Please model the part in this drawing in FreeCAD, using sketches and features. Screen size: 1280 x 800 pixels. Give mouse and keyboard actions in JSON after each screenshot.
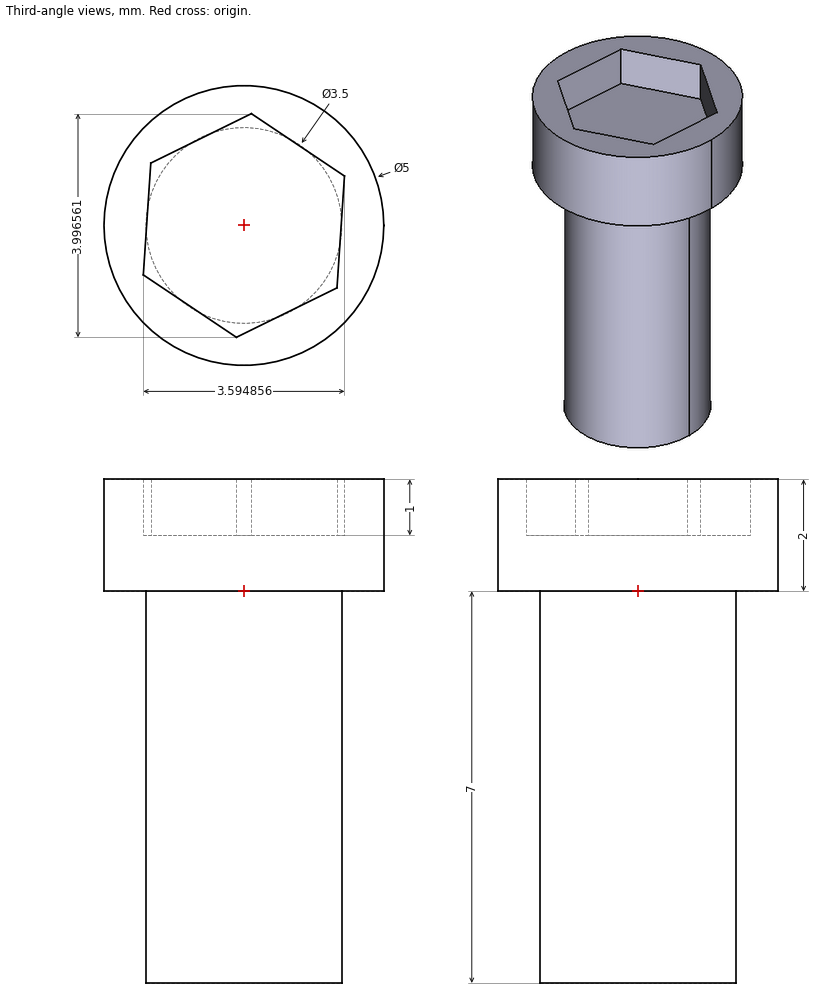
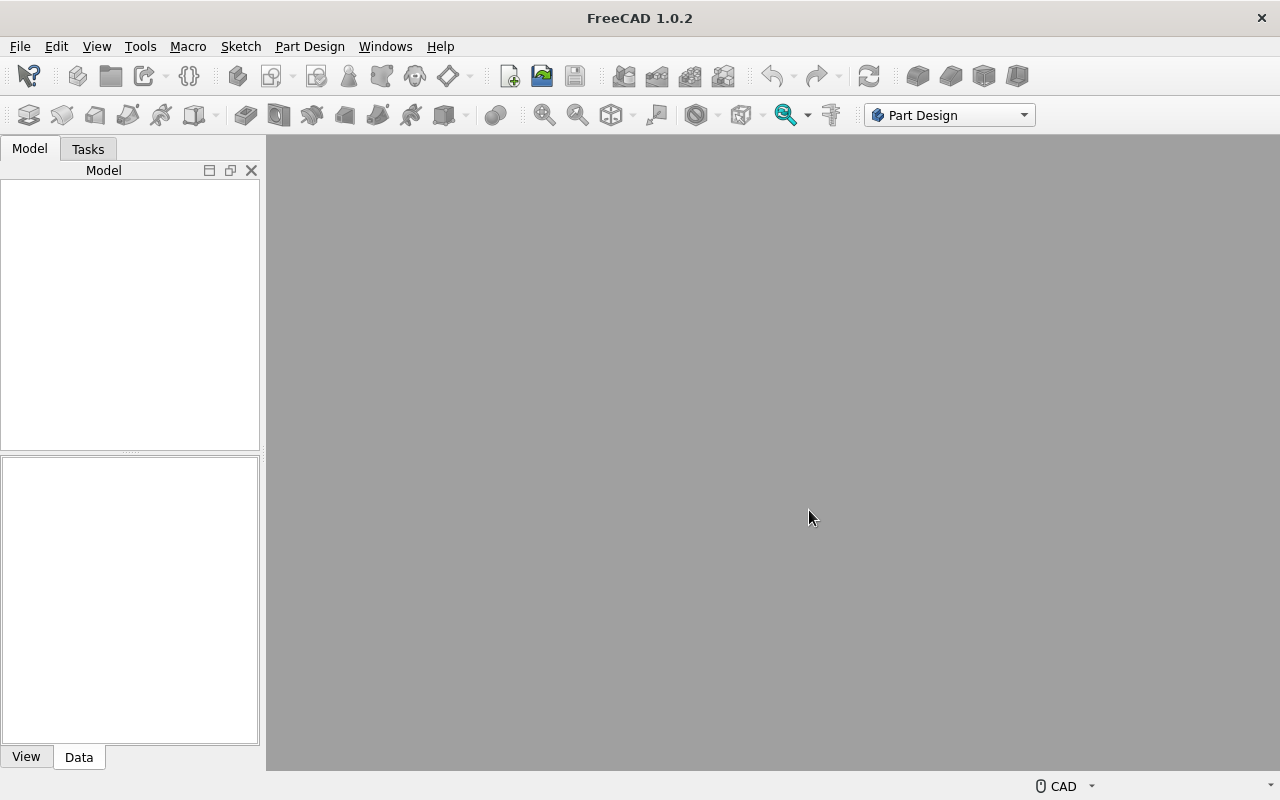
{"action": "left_click", "coordinate": [509, 76]}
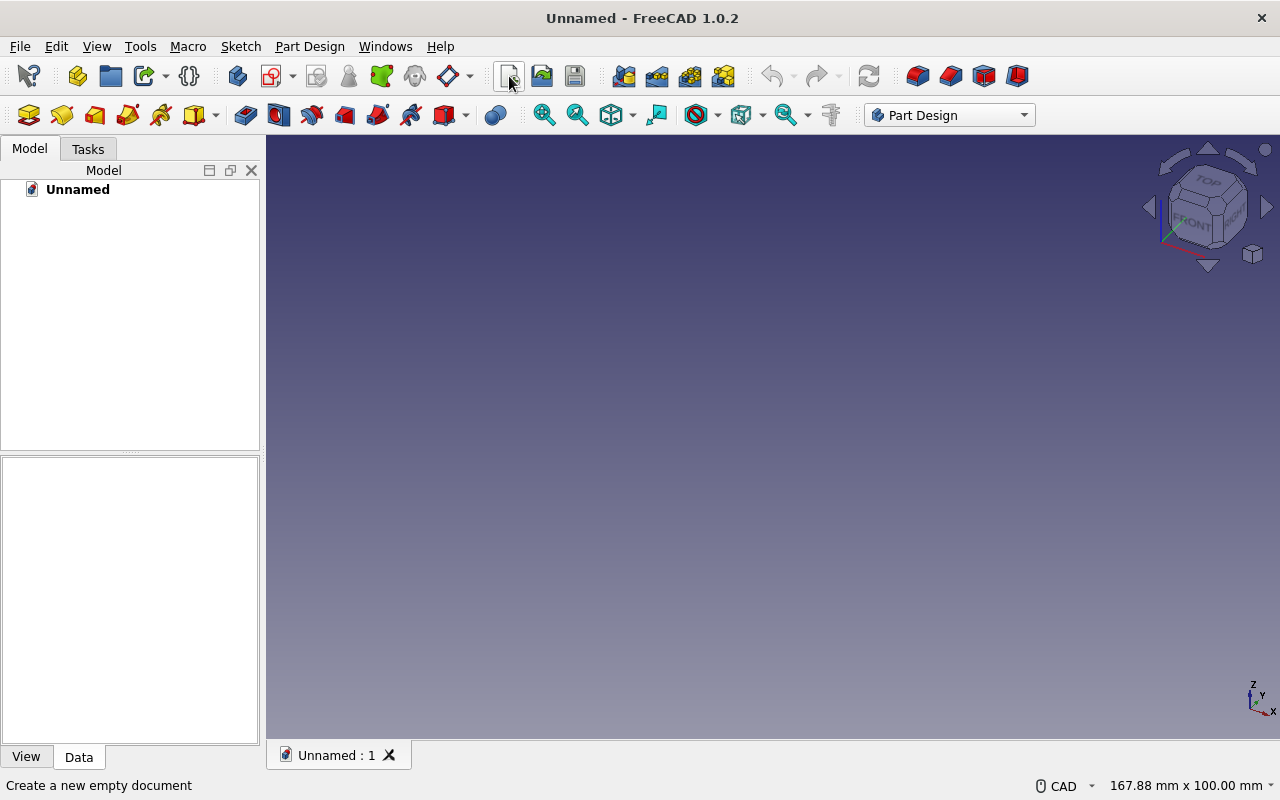
{"action": "left_click", "coordinate": [270, 76]}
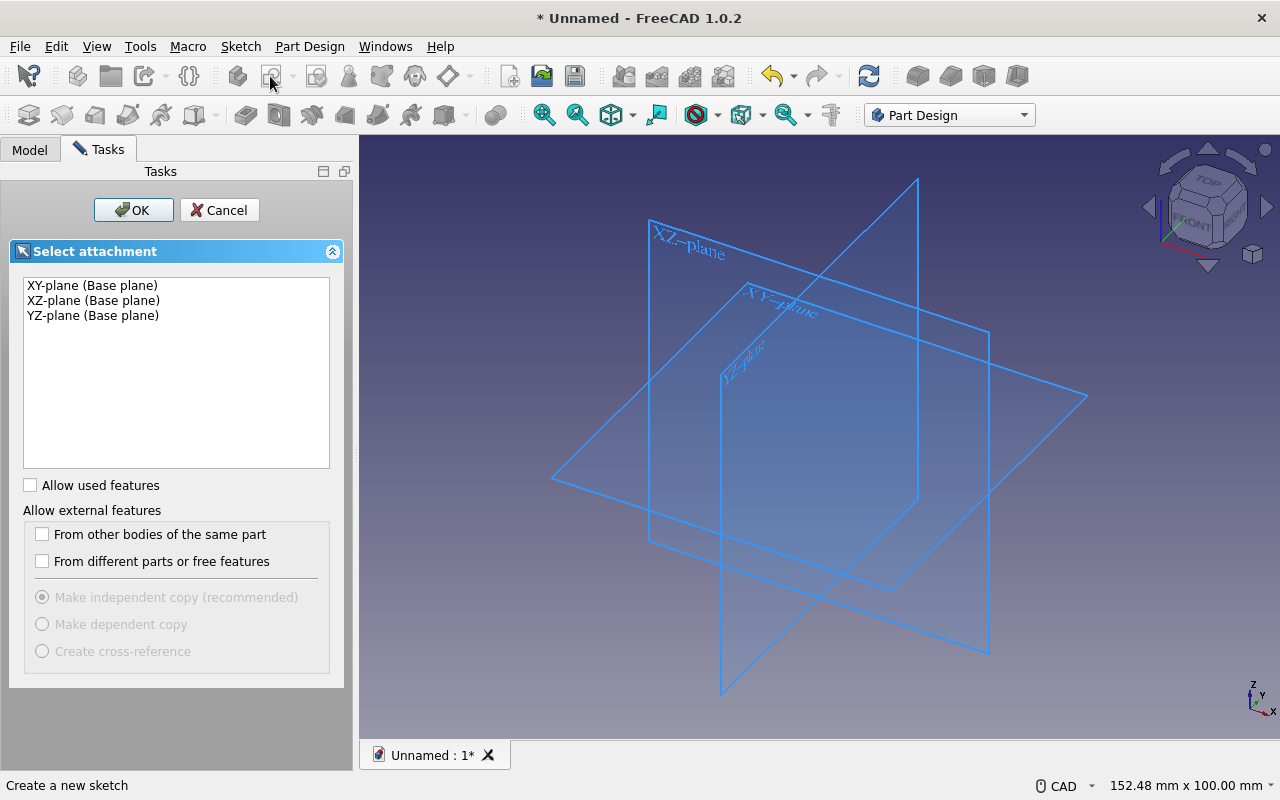
{"action": "left_click", "coordinate": [84, 286]}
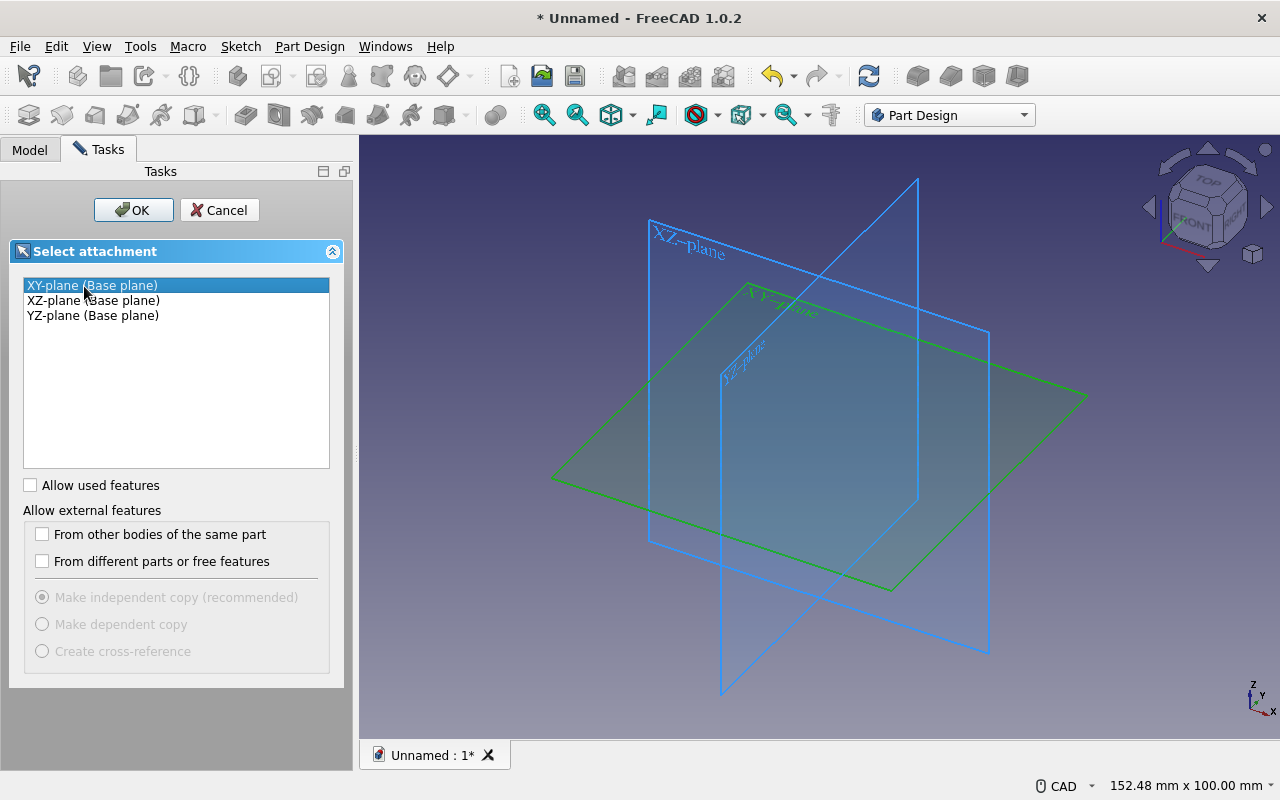
{"action": "left_click", "coordinate": [134, 210]}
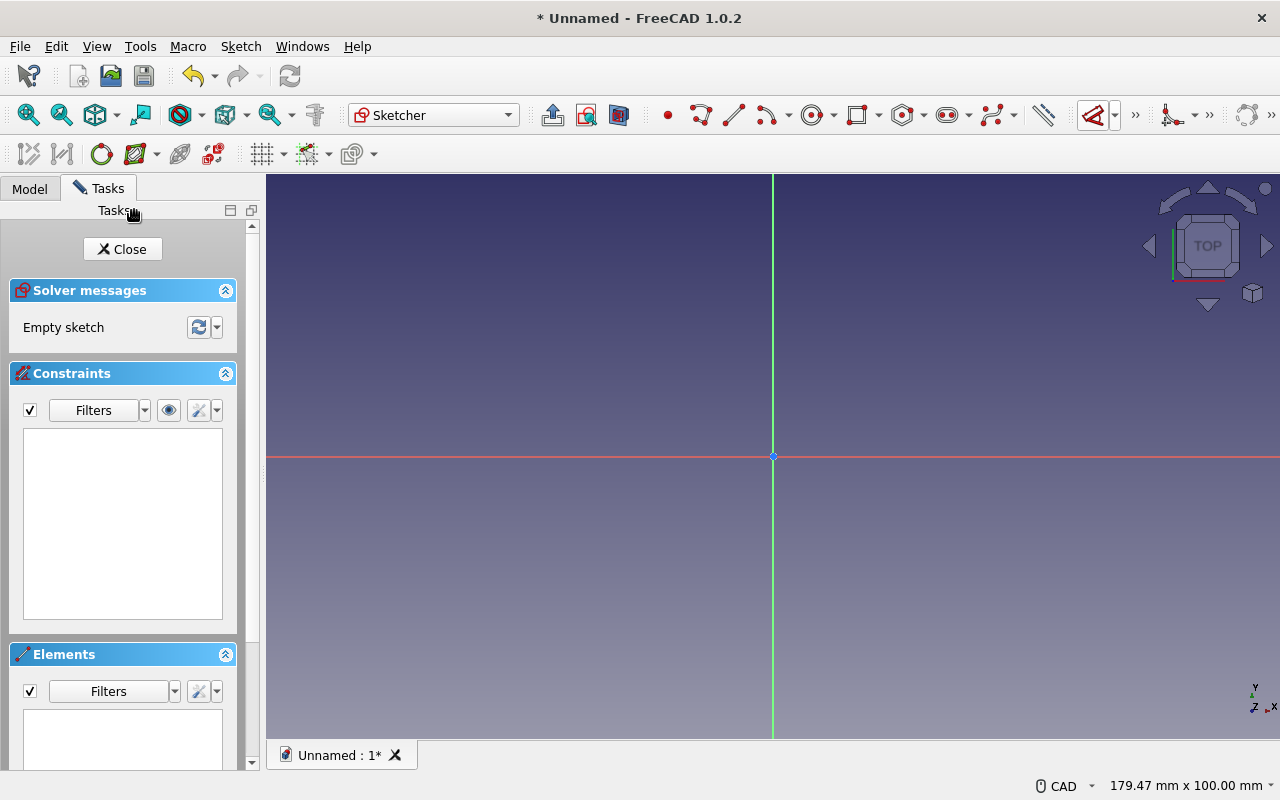
{"action": "scroll", "coordinate": [778, 456], "scroll_direction": "up", "scroll_amount": 13}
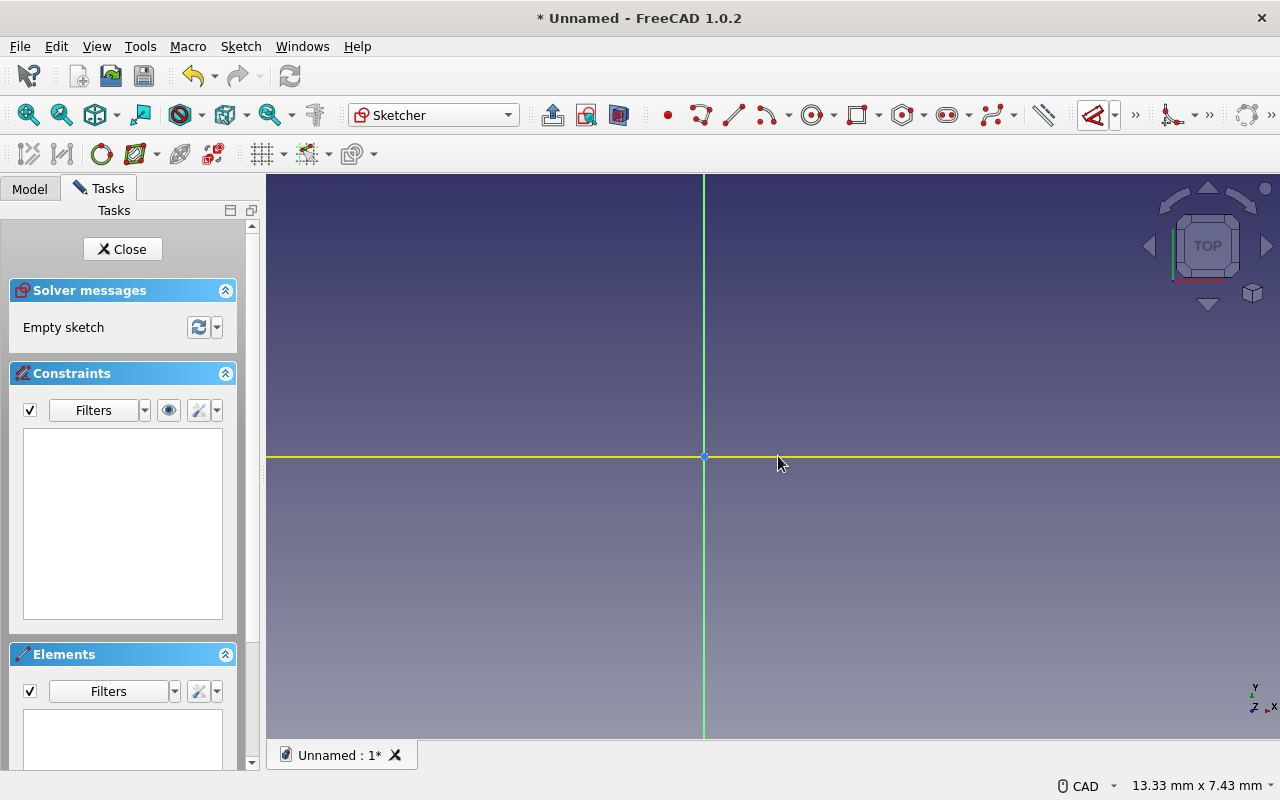
{"action": "left_click", "coordinate": [812, 116]}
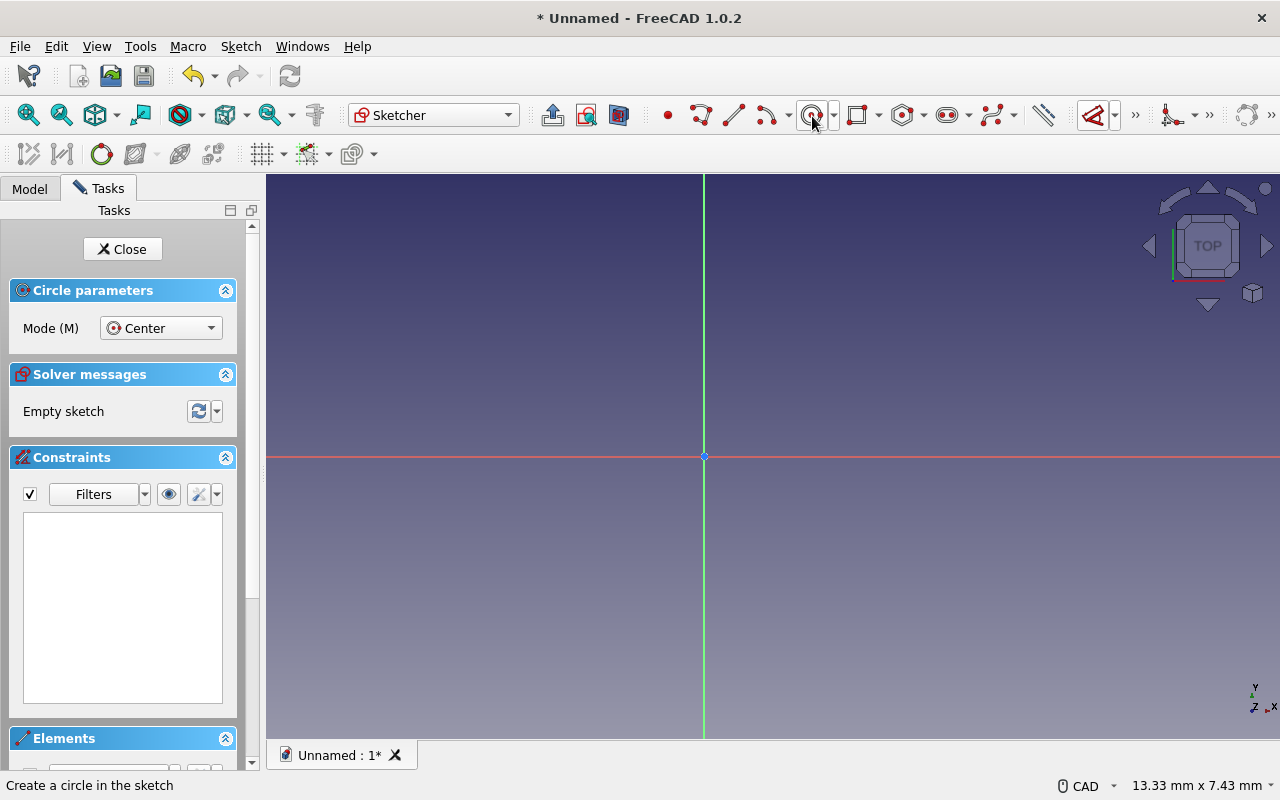
{"action": "left_click", "coordinate": [704, 456]}
{"action": "left_click", "coordinate": [839, 322]}
{"action": "key", "text": "Escape"}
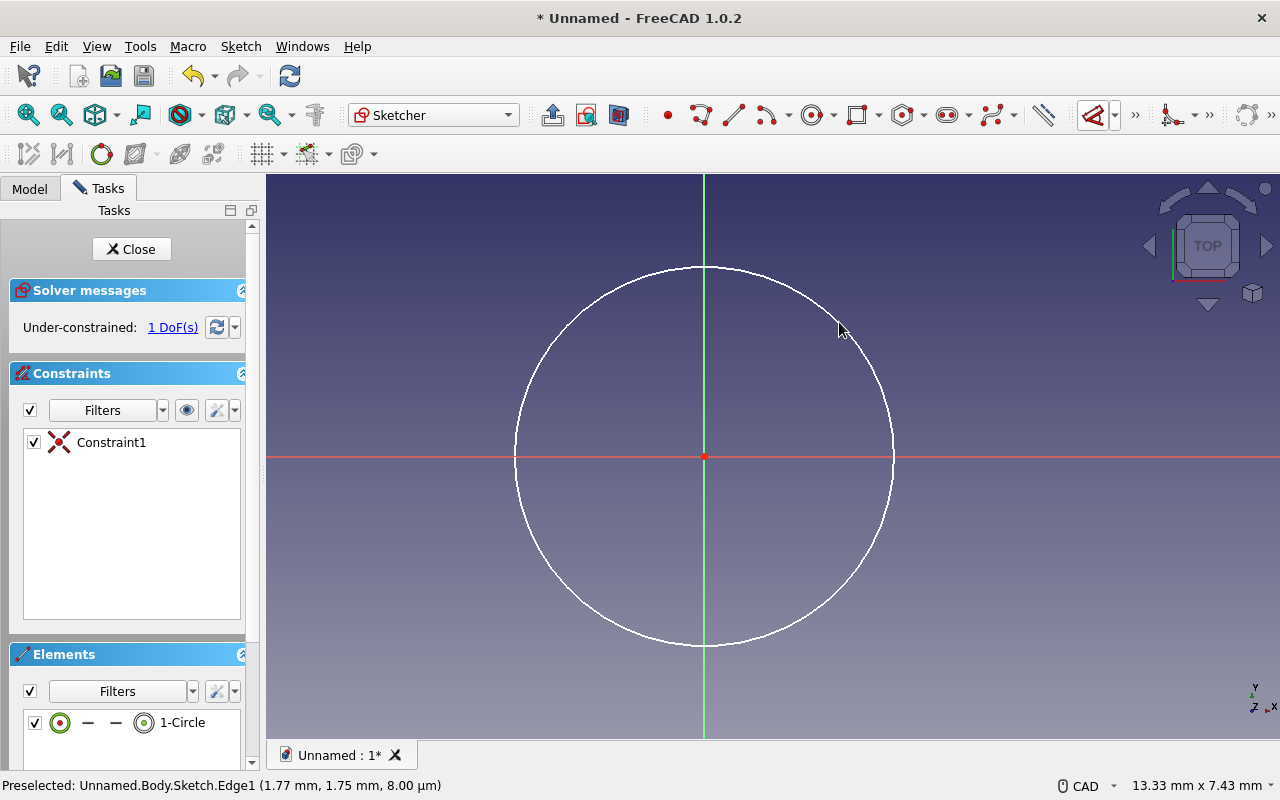
{"action": "left_click", "coordinate": [1092, 116]}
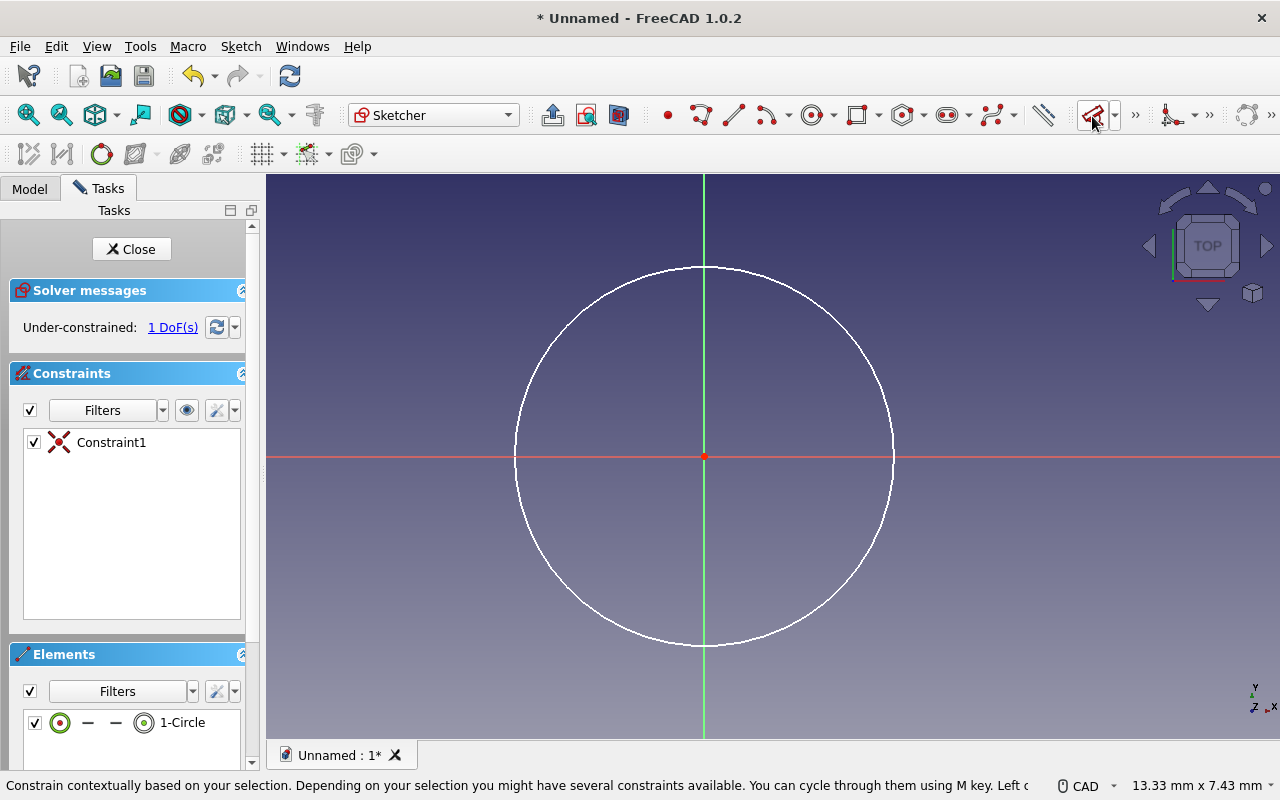
{"action": "left_click", "coordinate": [838, 322]}
{"action": "left_click", "coordinate": [861, 299]}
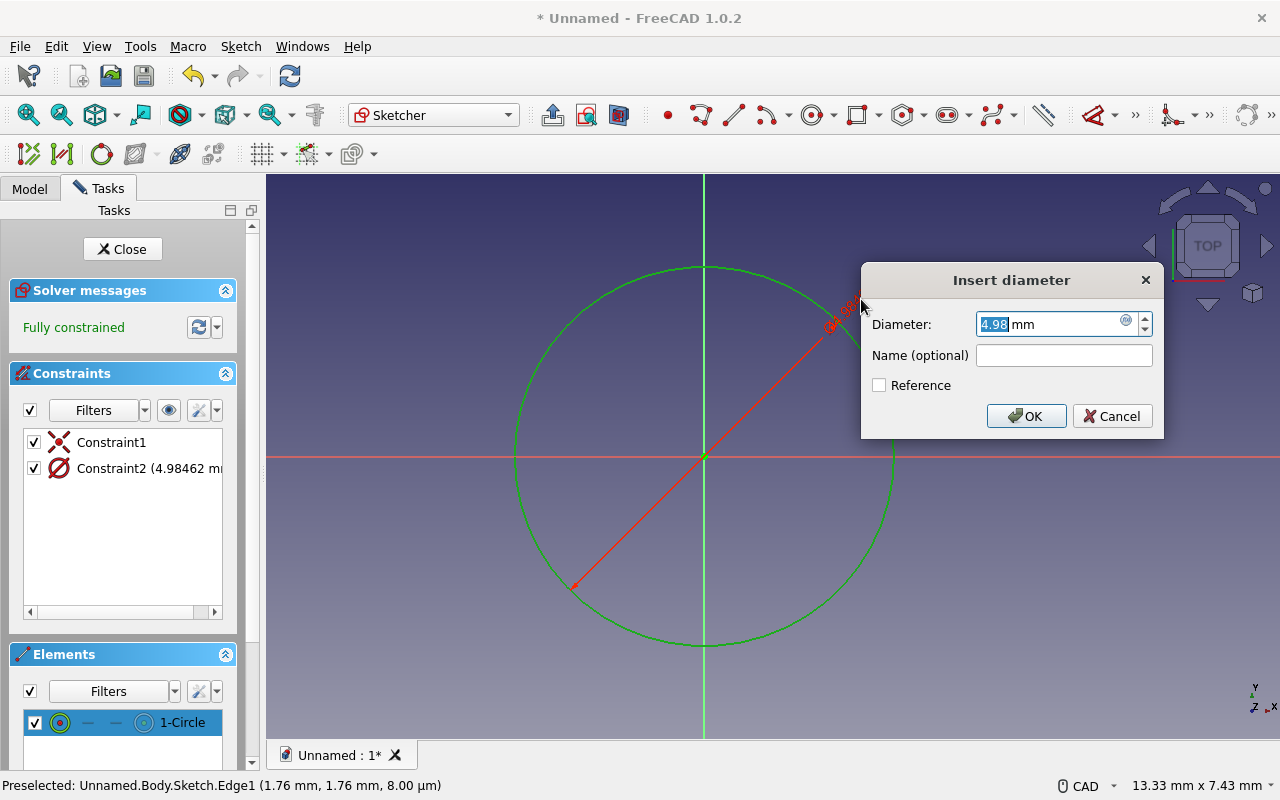
{"action": "type", "text": "5"}
{"action": "key", "text": "Return"}
{"action": "key", "text": "Escape"}